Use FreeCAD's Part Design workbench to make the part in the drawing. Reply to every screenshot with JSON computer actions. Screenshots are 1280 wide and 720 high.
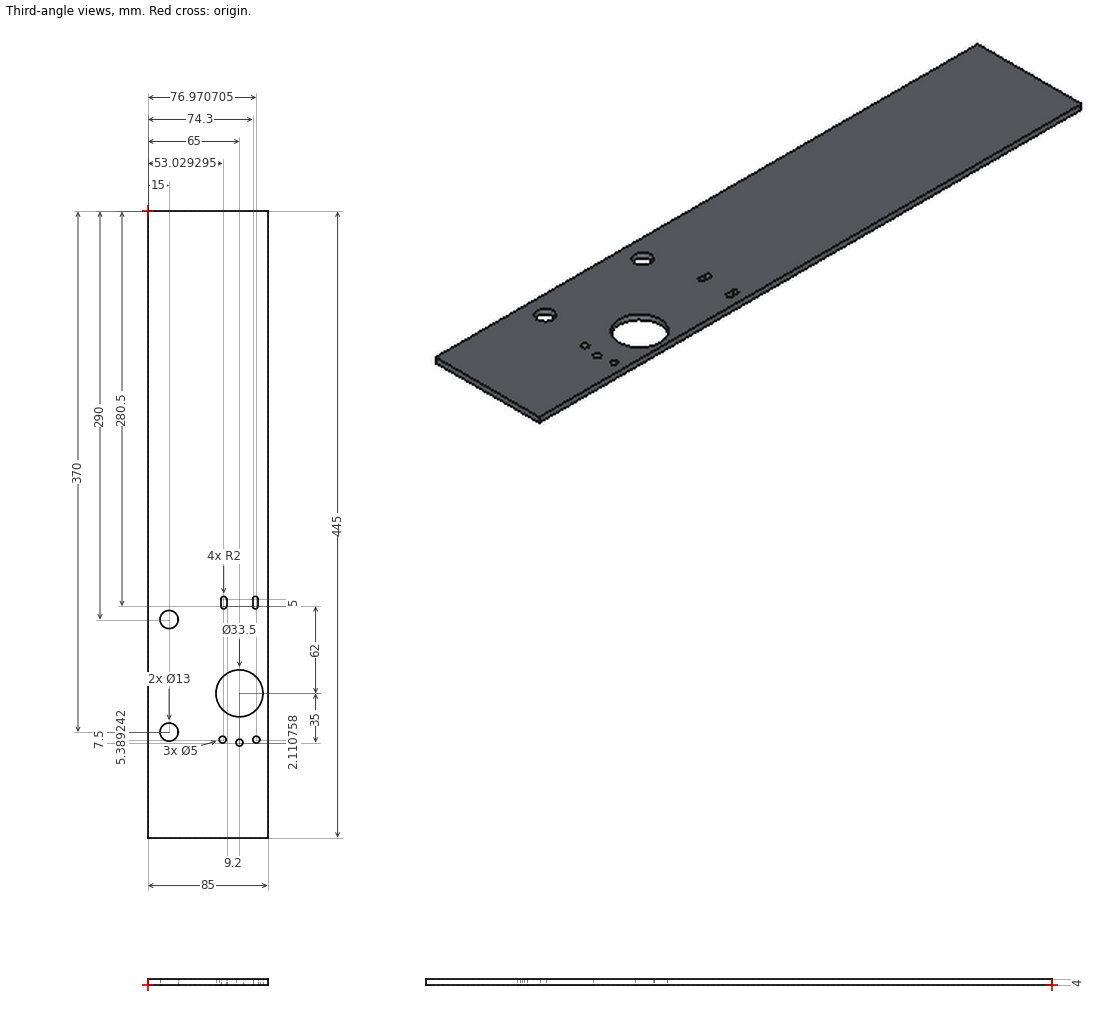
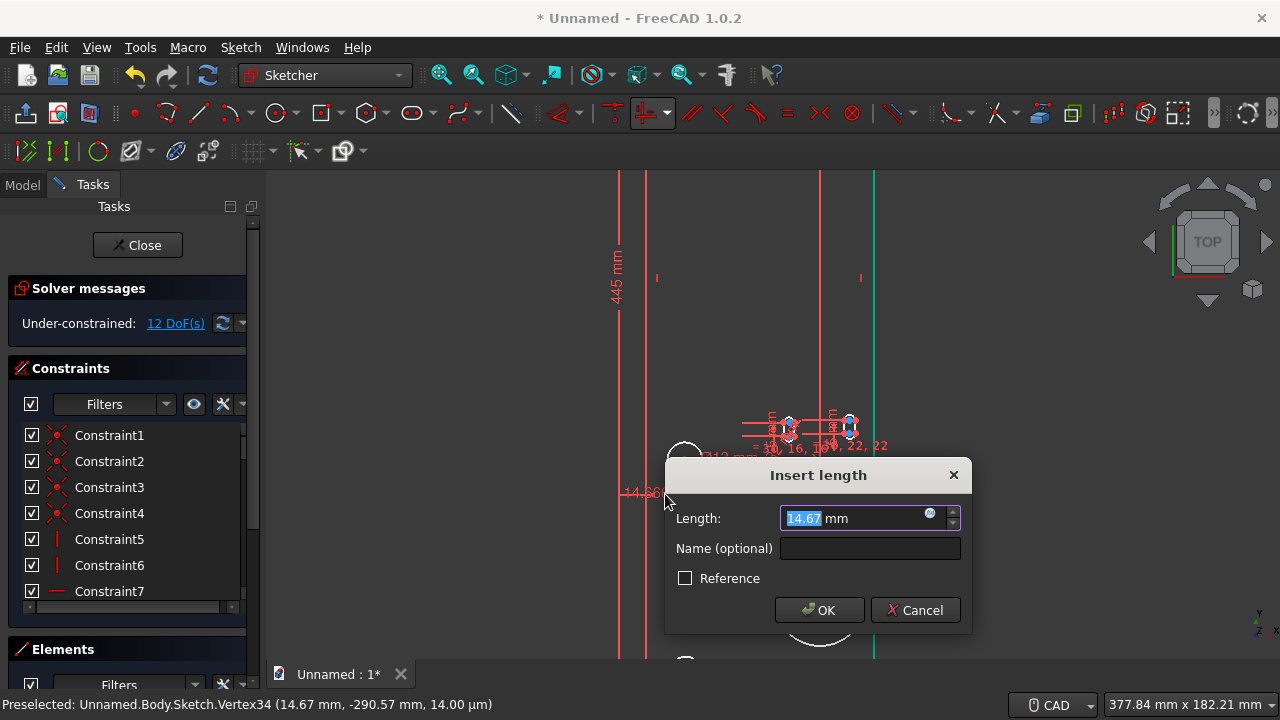
{"action": "type", "text": "15"}
{"action": "key", "text": "Return"}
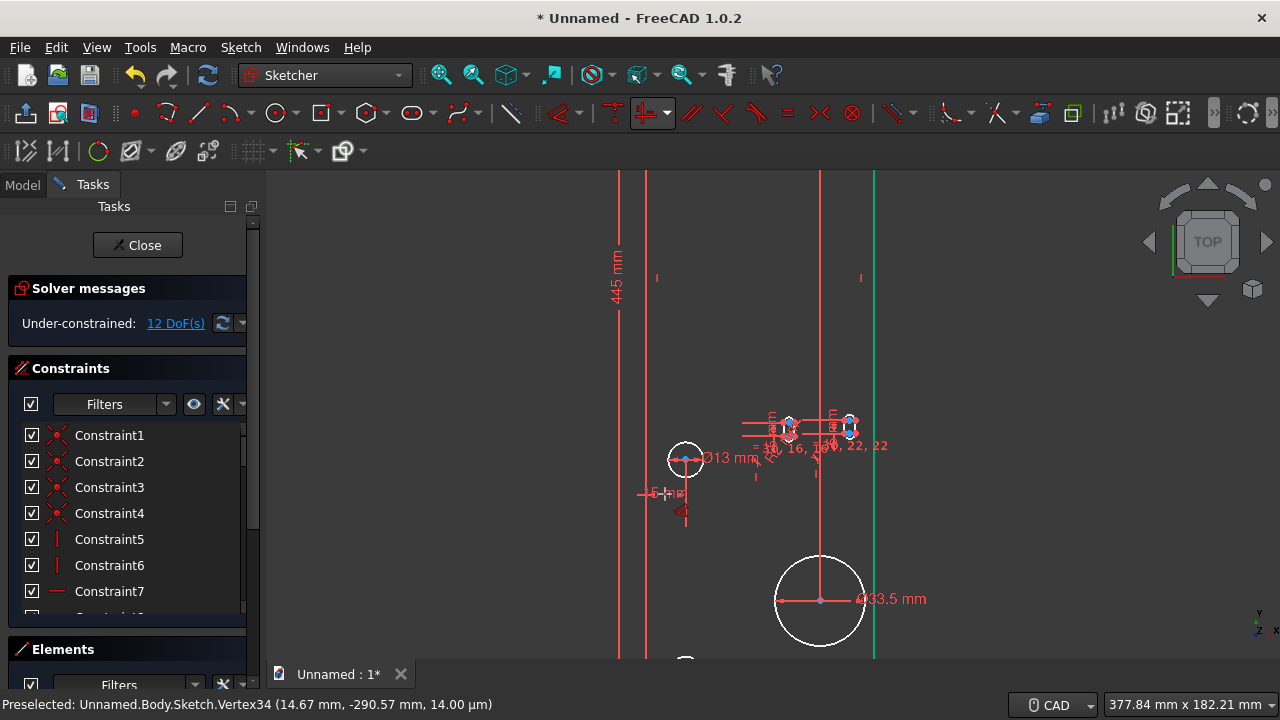
{"action": "scroll", "coordinate": [686, 459], "scroll_direction": "down", "scroll_amount": 7}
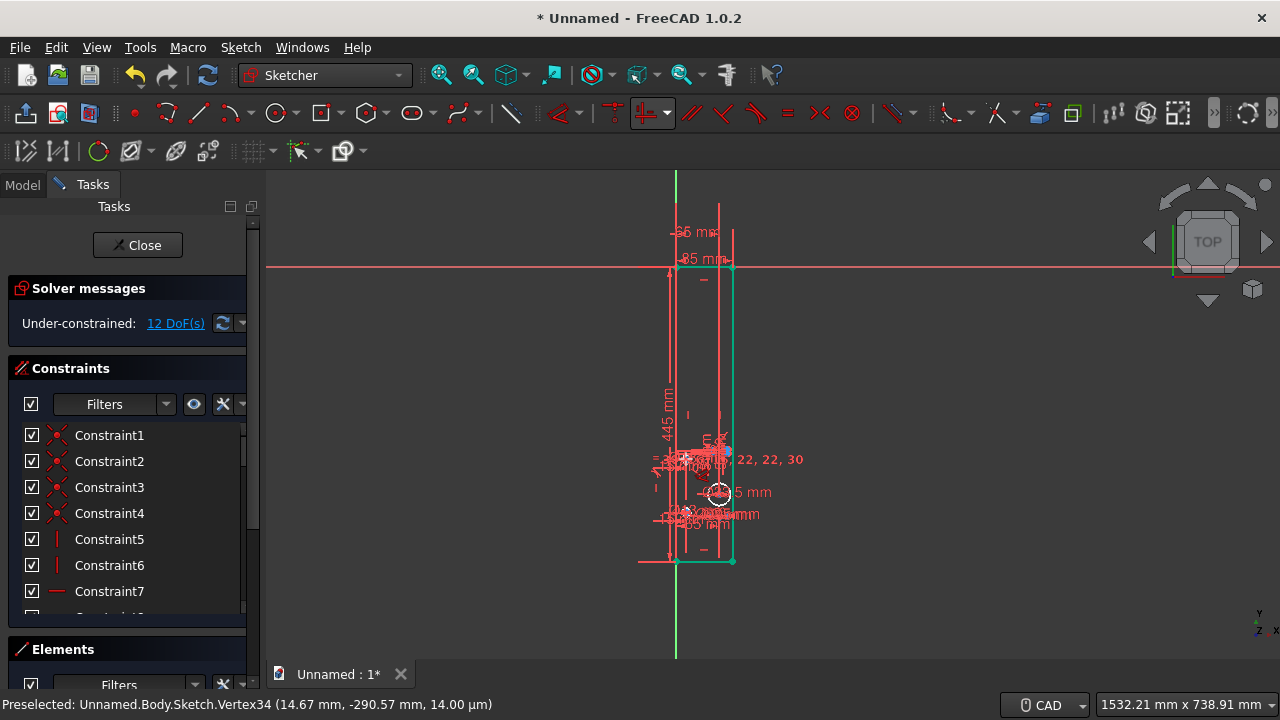
{"action": "left_click", "coordinate": [686, 513]}
{"action": "left_click", "coordinate": [642, 390]}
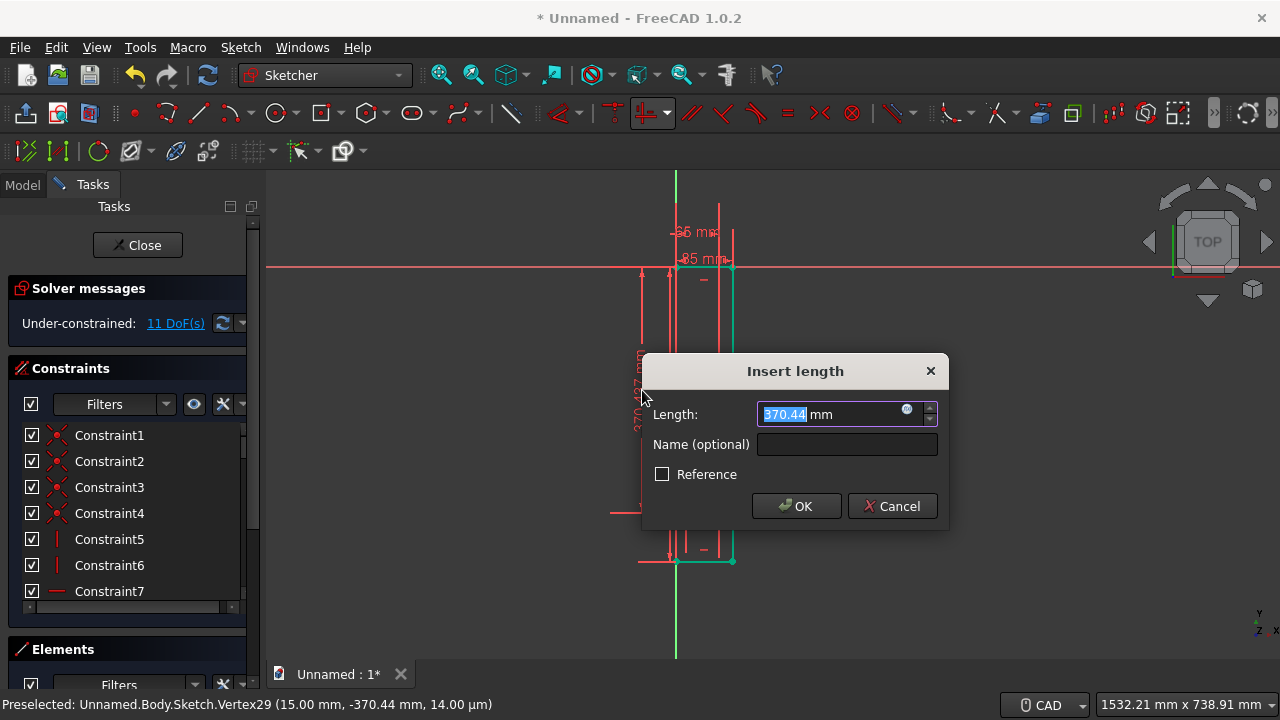
{"action": "type", "text": "370"}
{"action": "key", "text": "Return"}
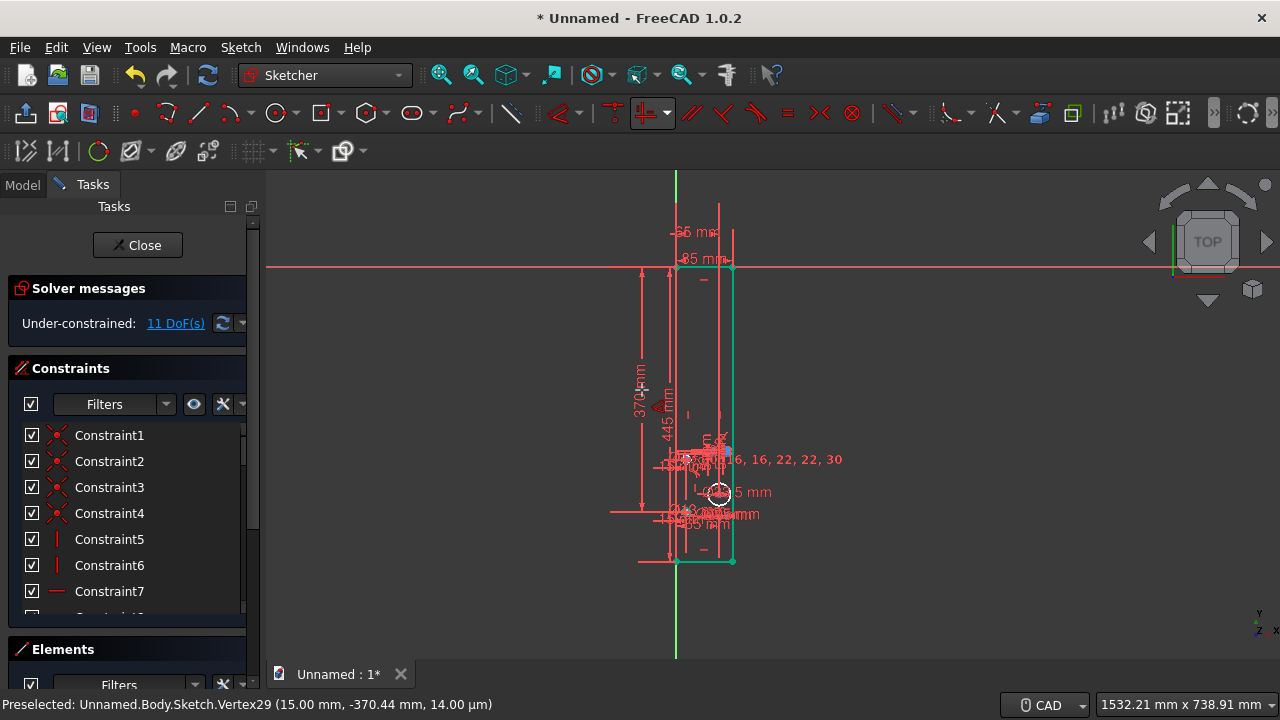
{"action": "left_click", "coordinate": [686, 460]}
{"action": "left_click", "coordinate": [642, 364]}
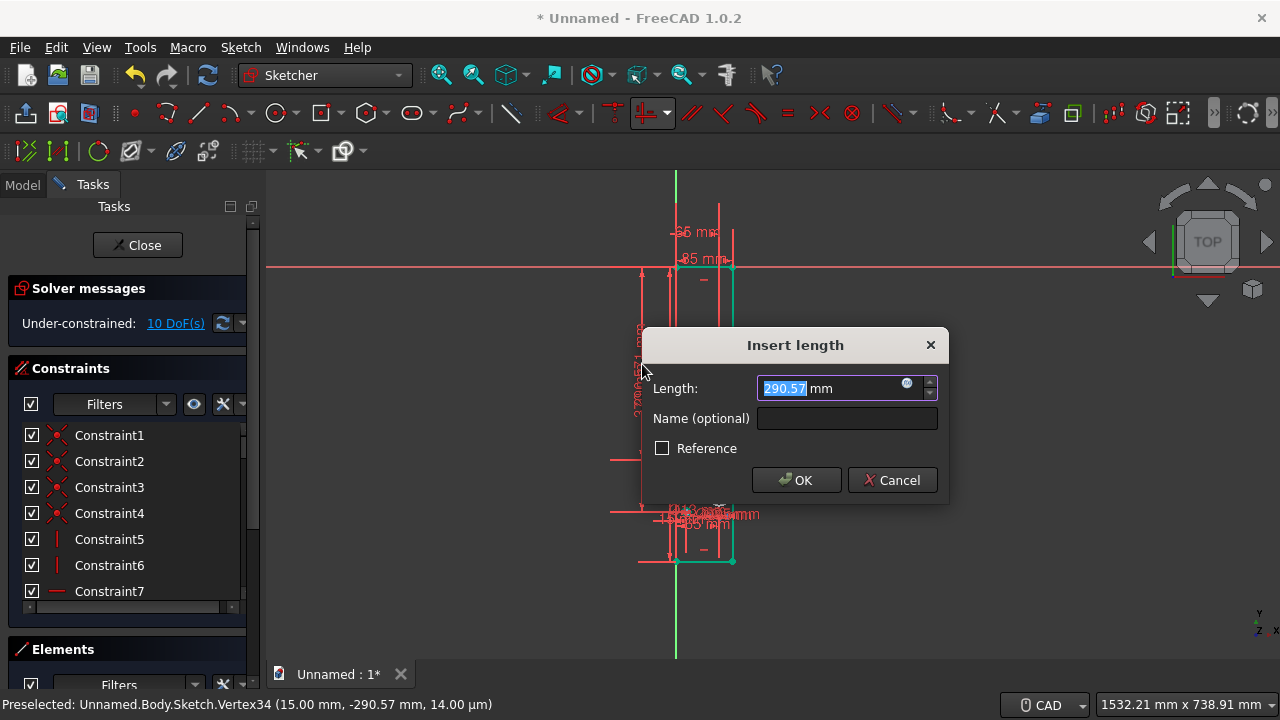
{"action": "type", "text": "290"}
{"action": "key", "text": "Return"}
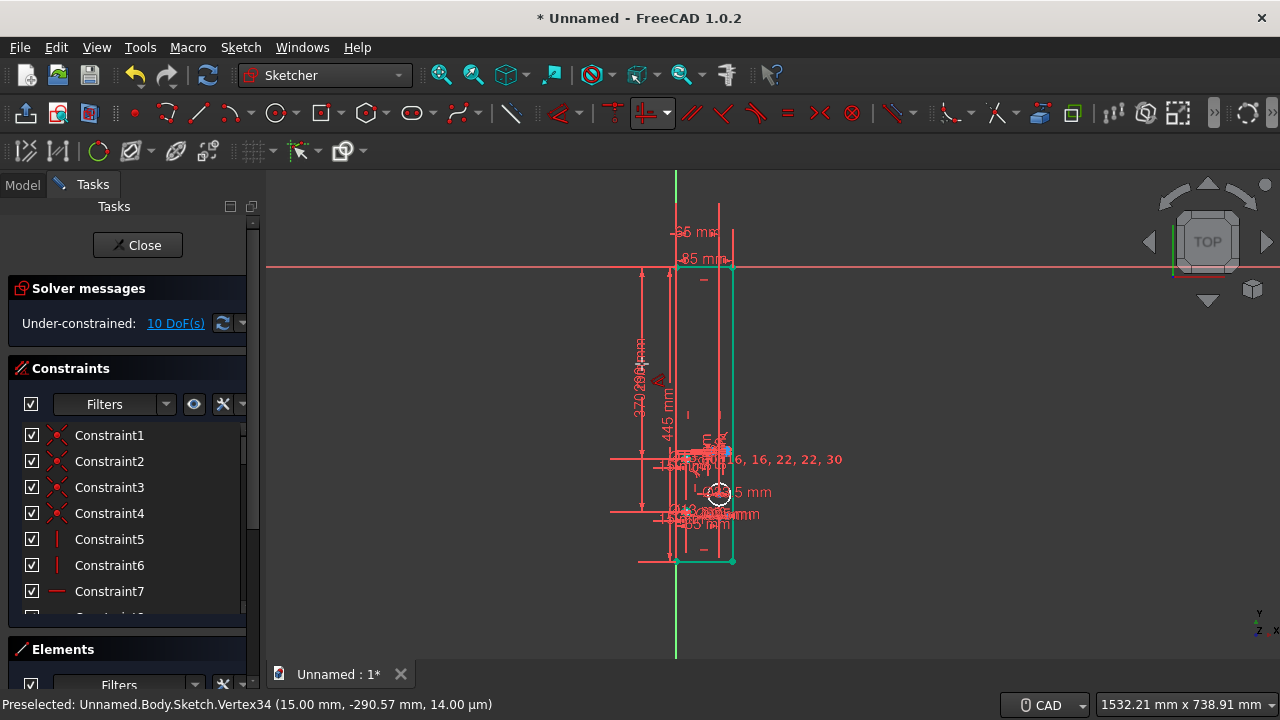
{"action": "scroll", "coordinate": [719, 517], "scroll_direction": "up", "scroll_amount": 3}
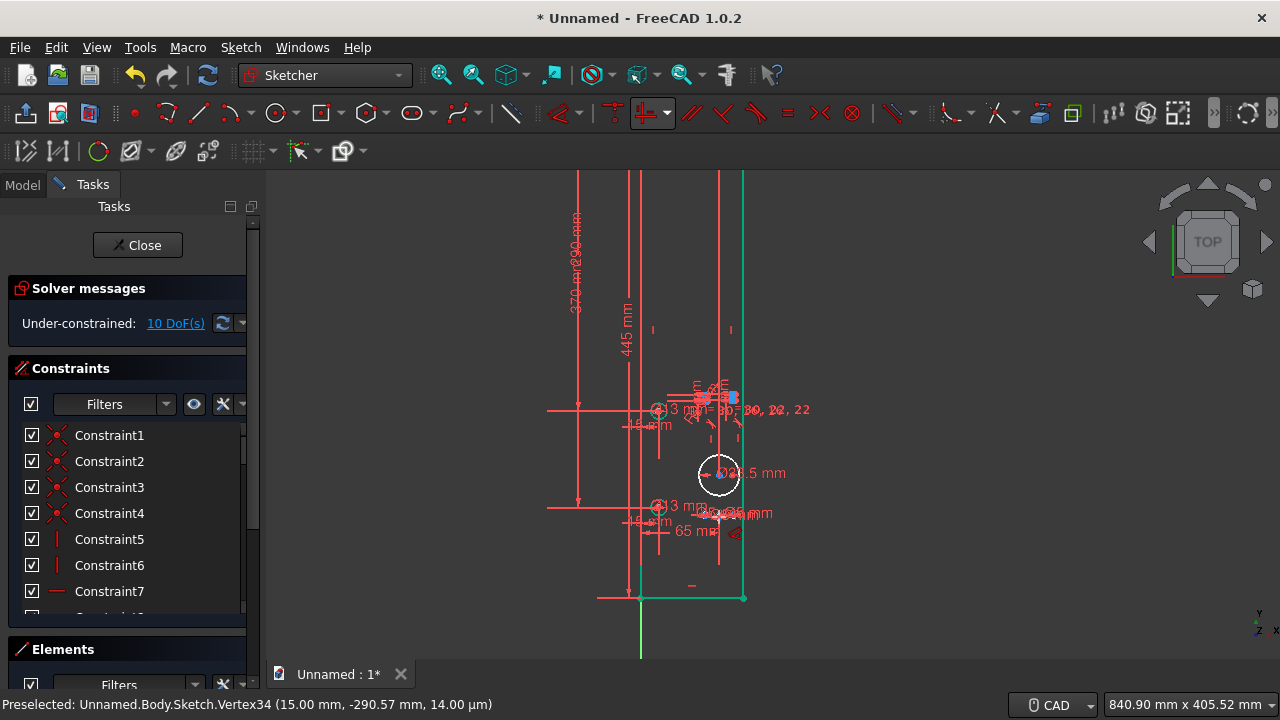
{"action": "left_click", "coordinate": [719, 517]}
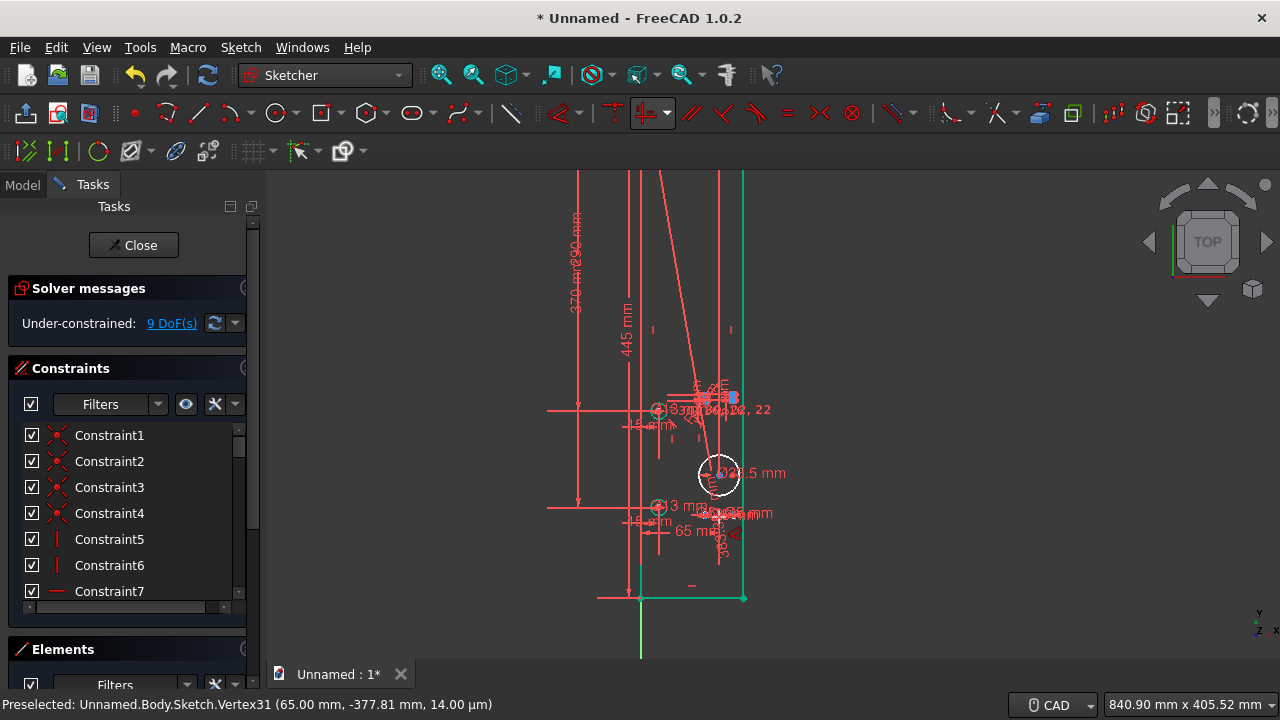
{"action": "left_click", "coordinate": [719, 475]}
{"action": "left_click", "coordinate": [685, 496]}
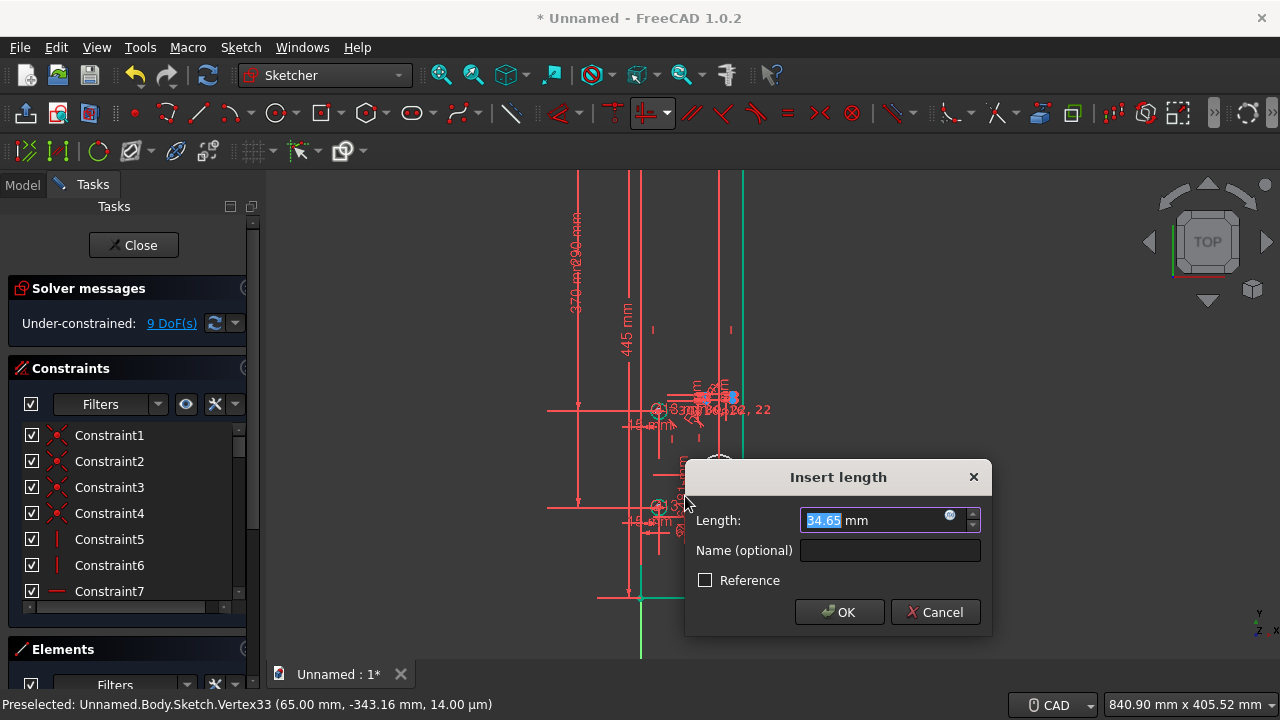
{"action": "type", "text": "35"}
{"action": "key", "text": "Return"}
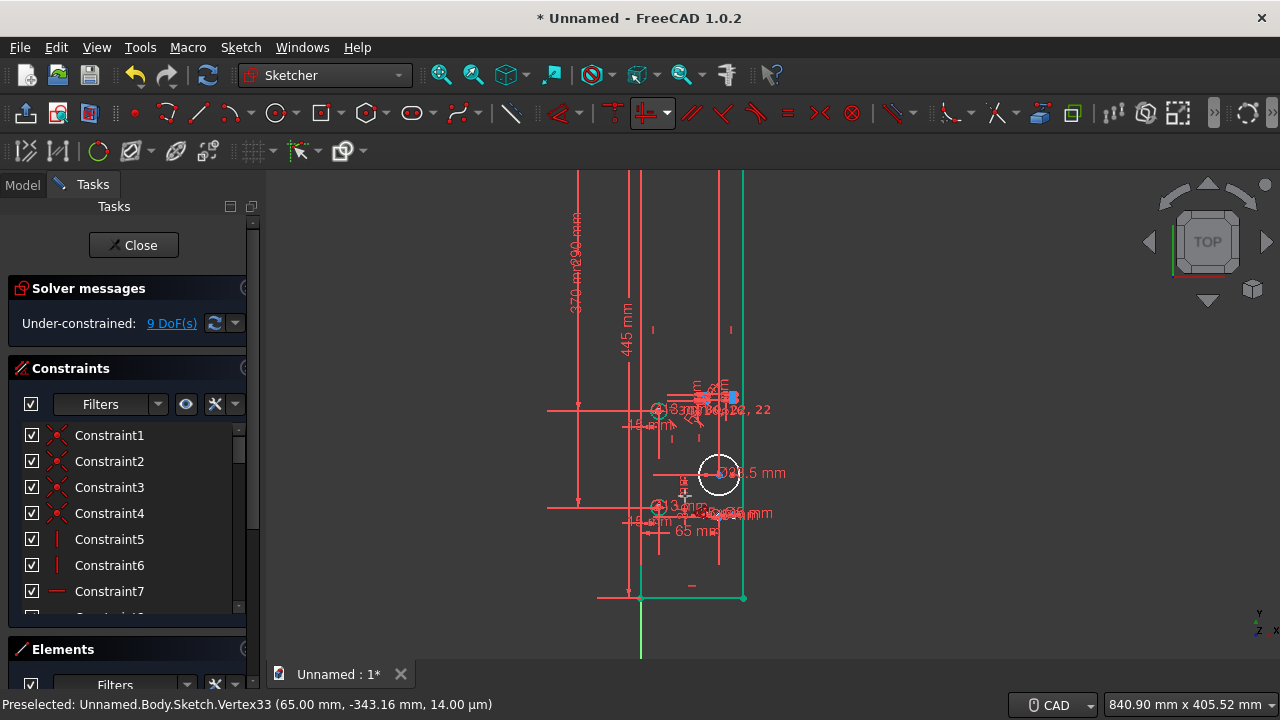
{"action": "scroll", "coordinate": [708, 401], "scroll_direction": "up", "scroll_amount": 9}